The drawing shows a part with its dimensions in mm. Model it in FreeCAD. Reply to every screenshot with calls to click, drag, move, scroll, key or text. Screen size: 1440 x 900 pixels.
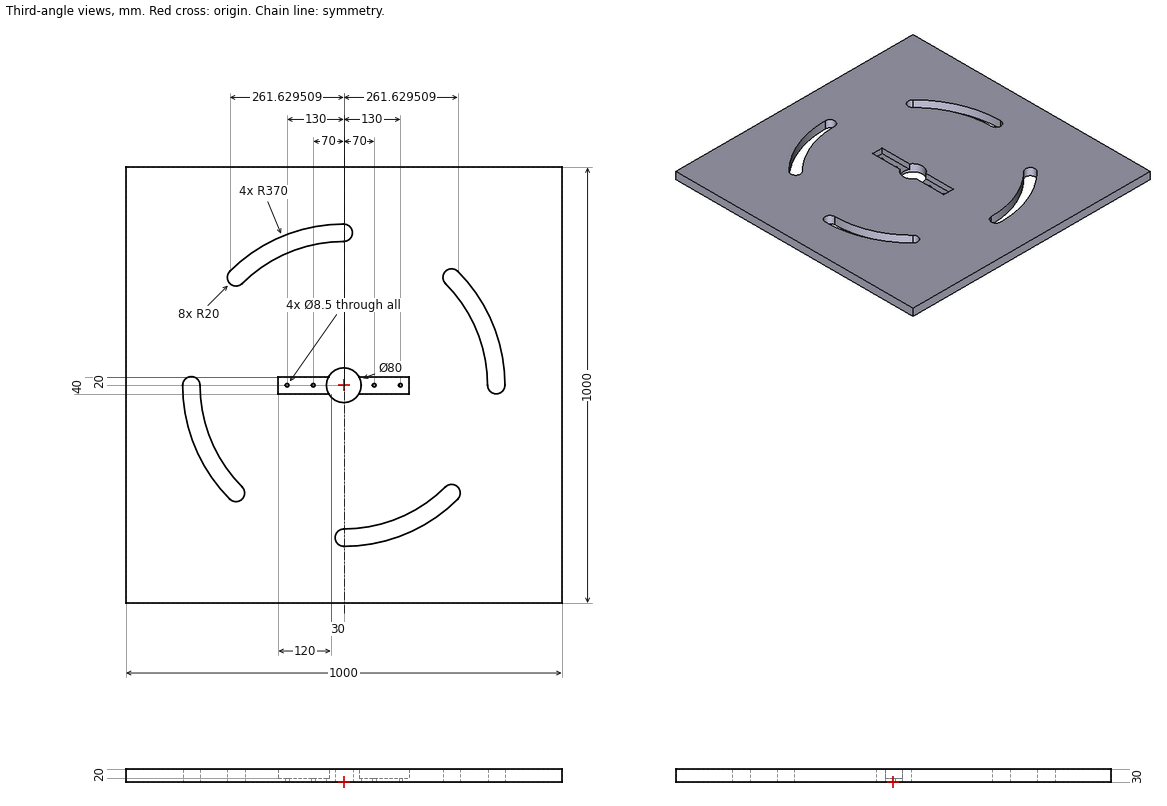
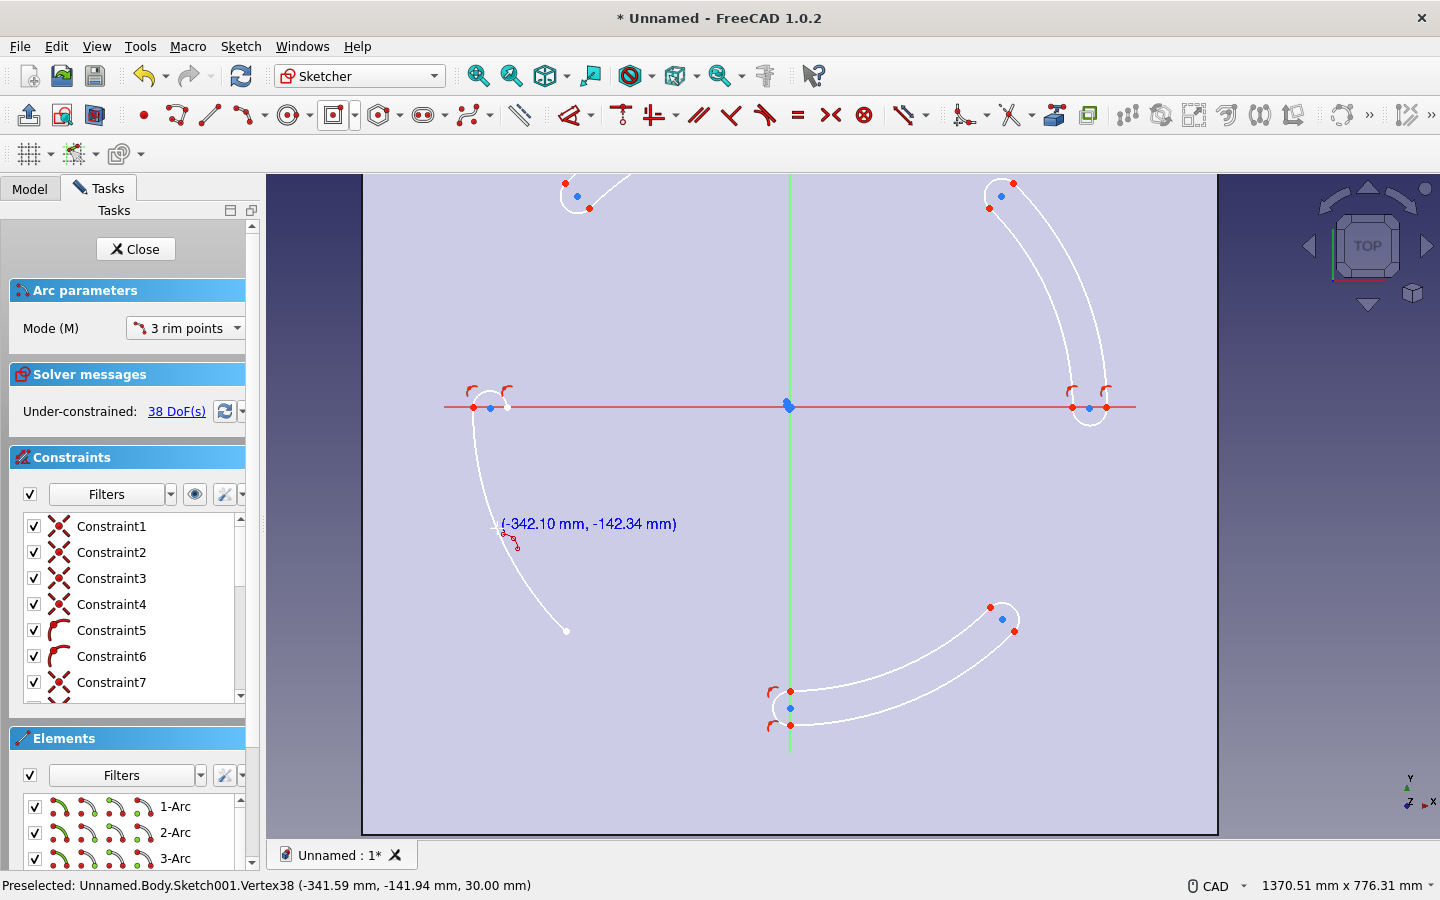
click(566, 632)
click(590, 607)
click(590, 631)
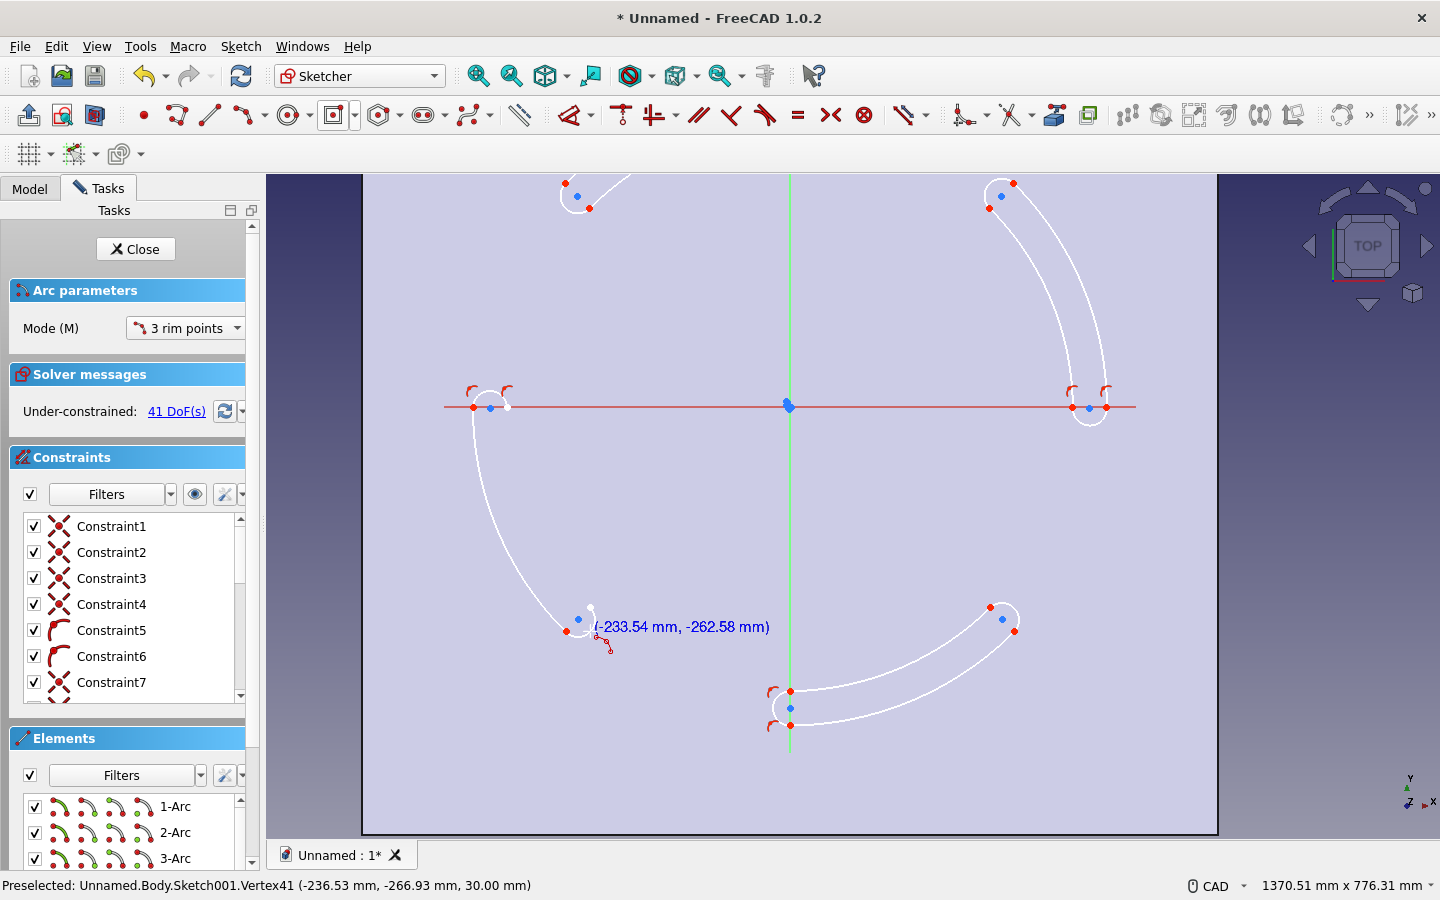
click(590, 608)
click(507, 407)
click(529, 515)
key(Escape)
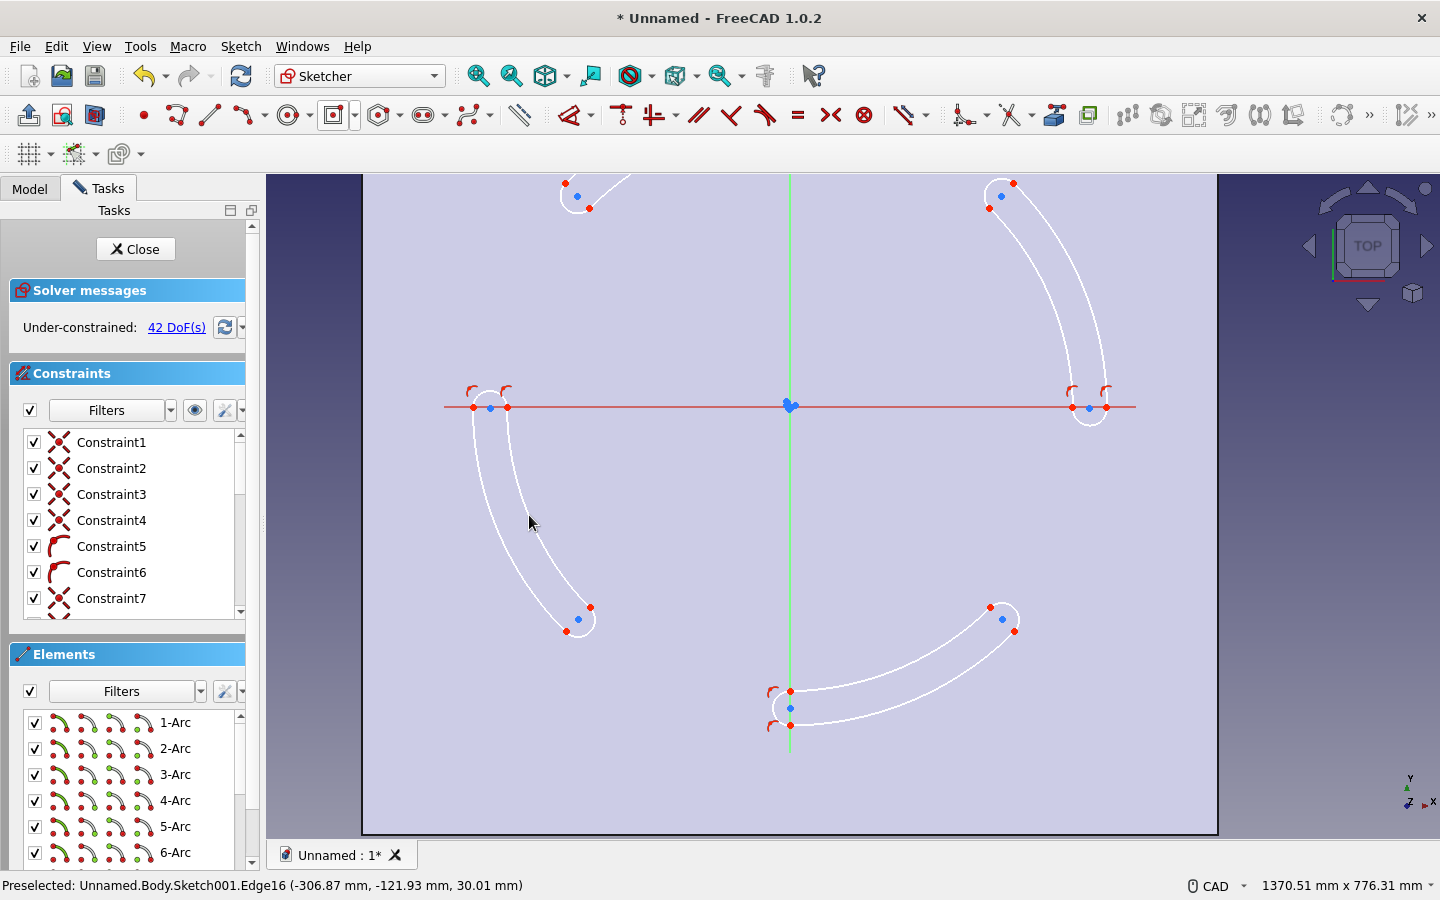
scroll(773, 709, down, 2)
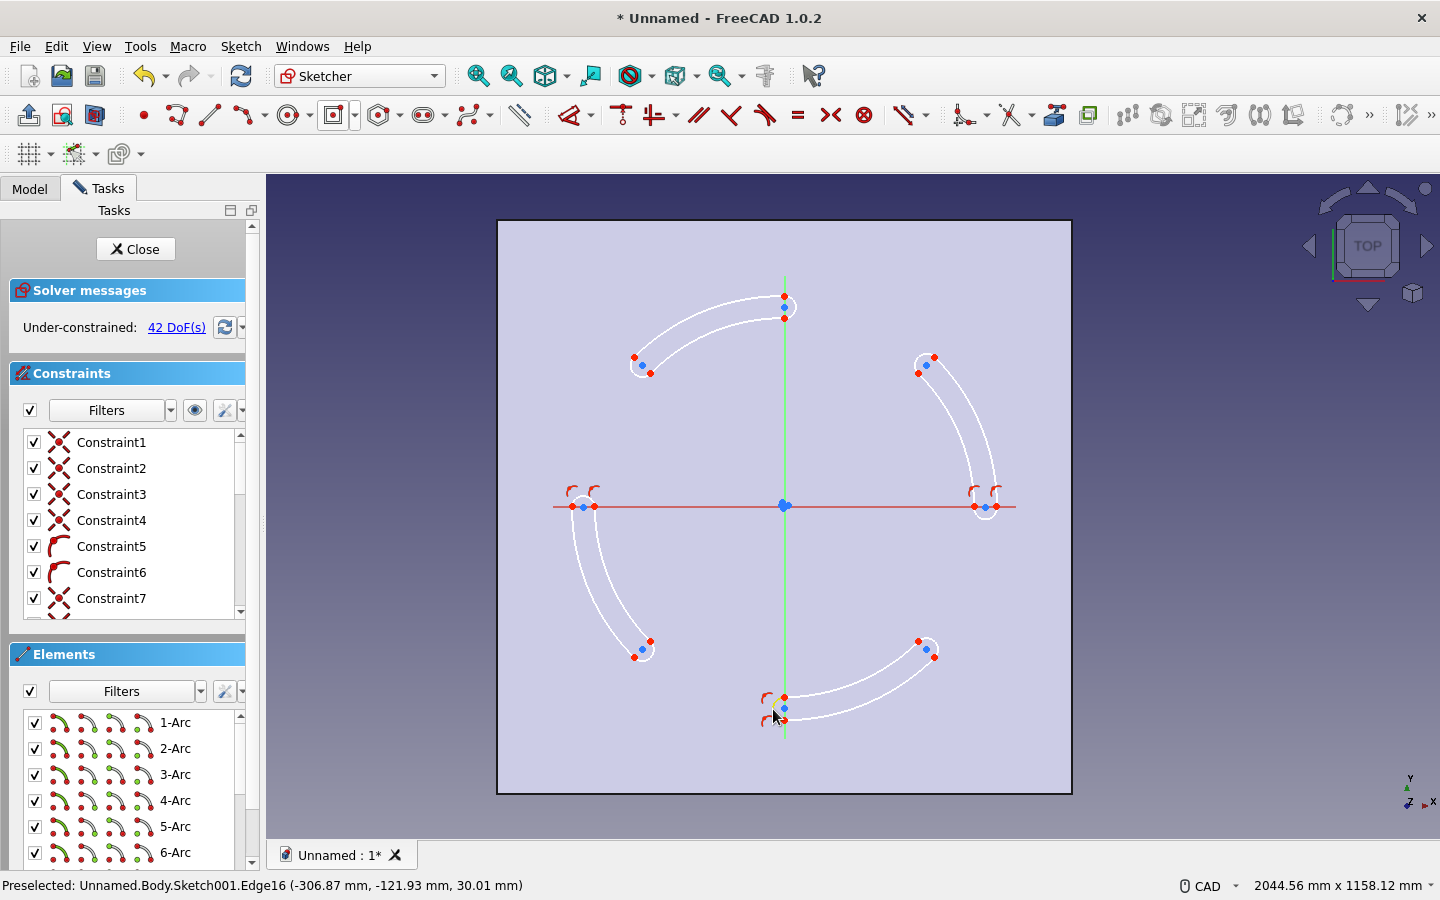
scroll(794, 314, up, 3)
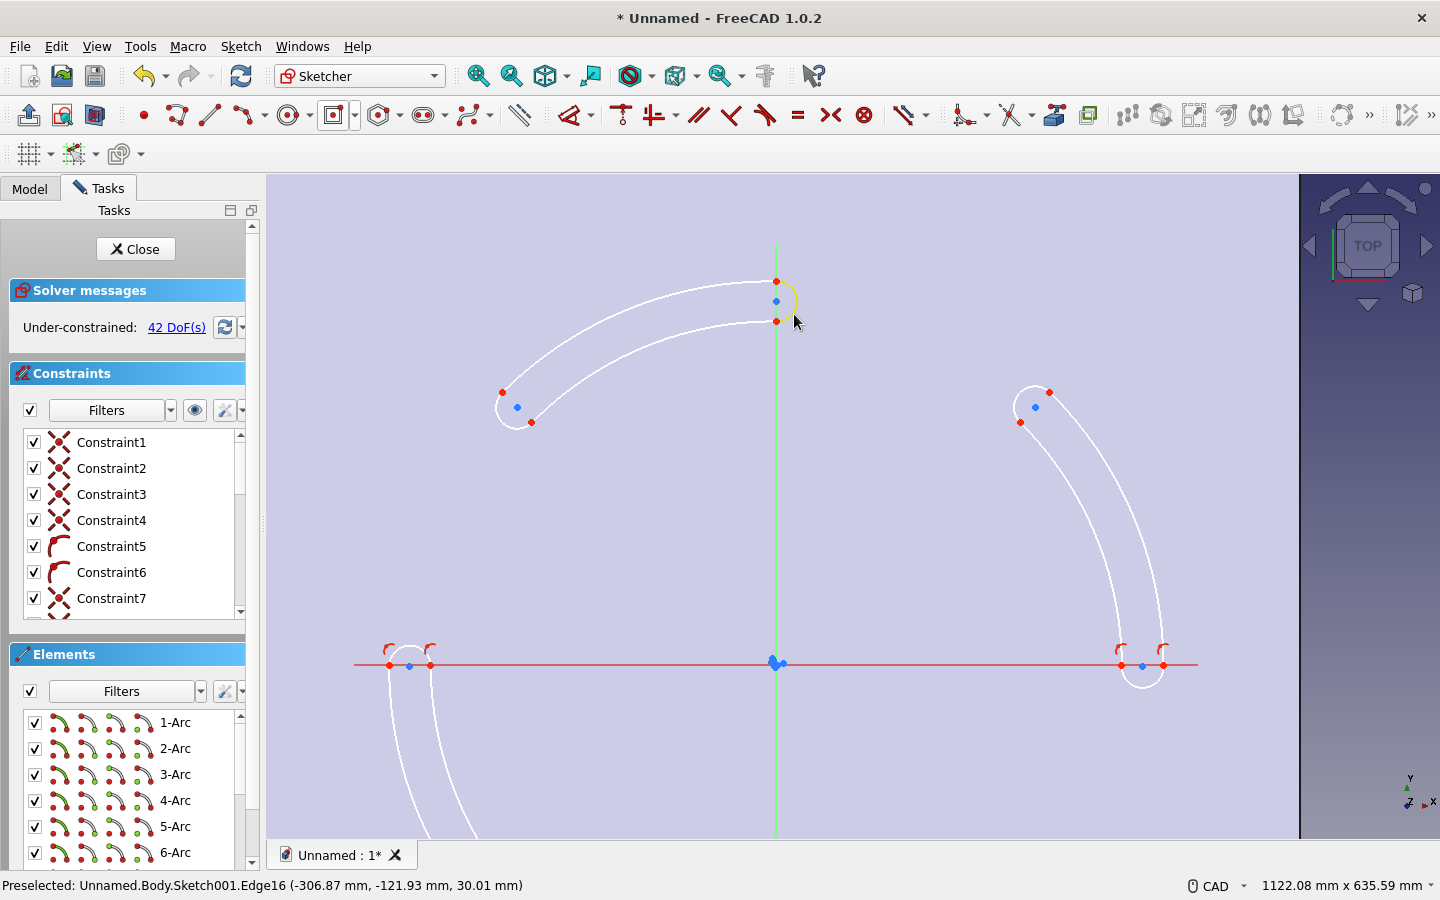
click(793, 313)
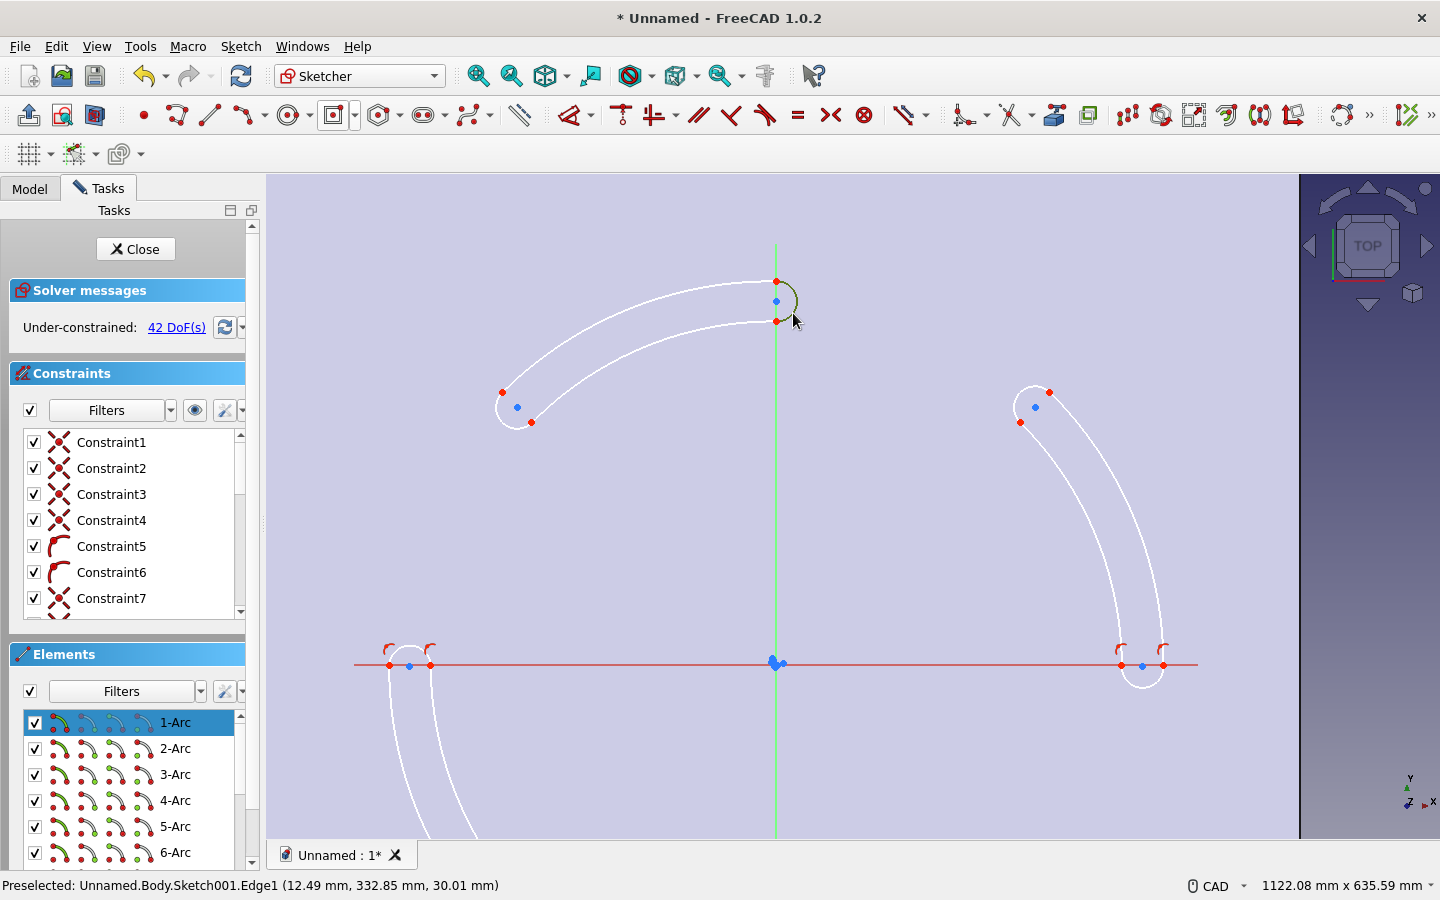
click(686, 291)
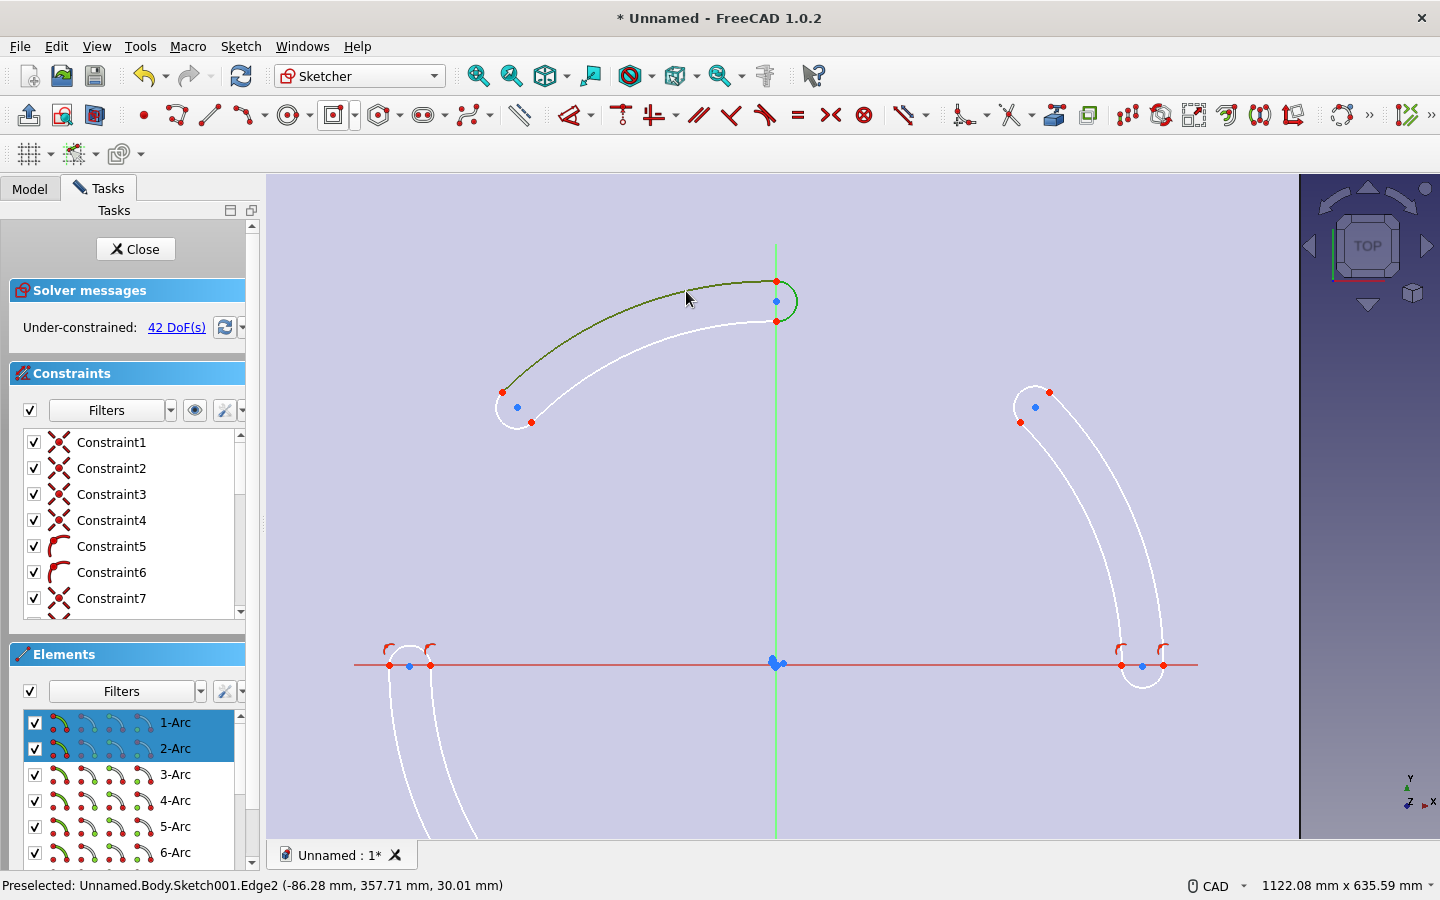
key(t)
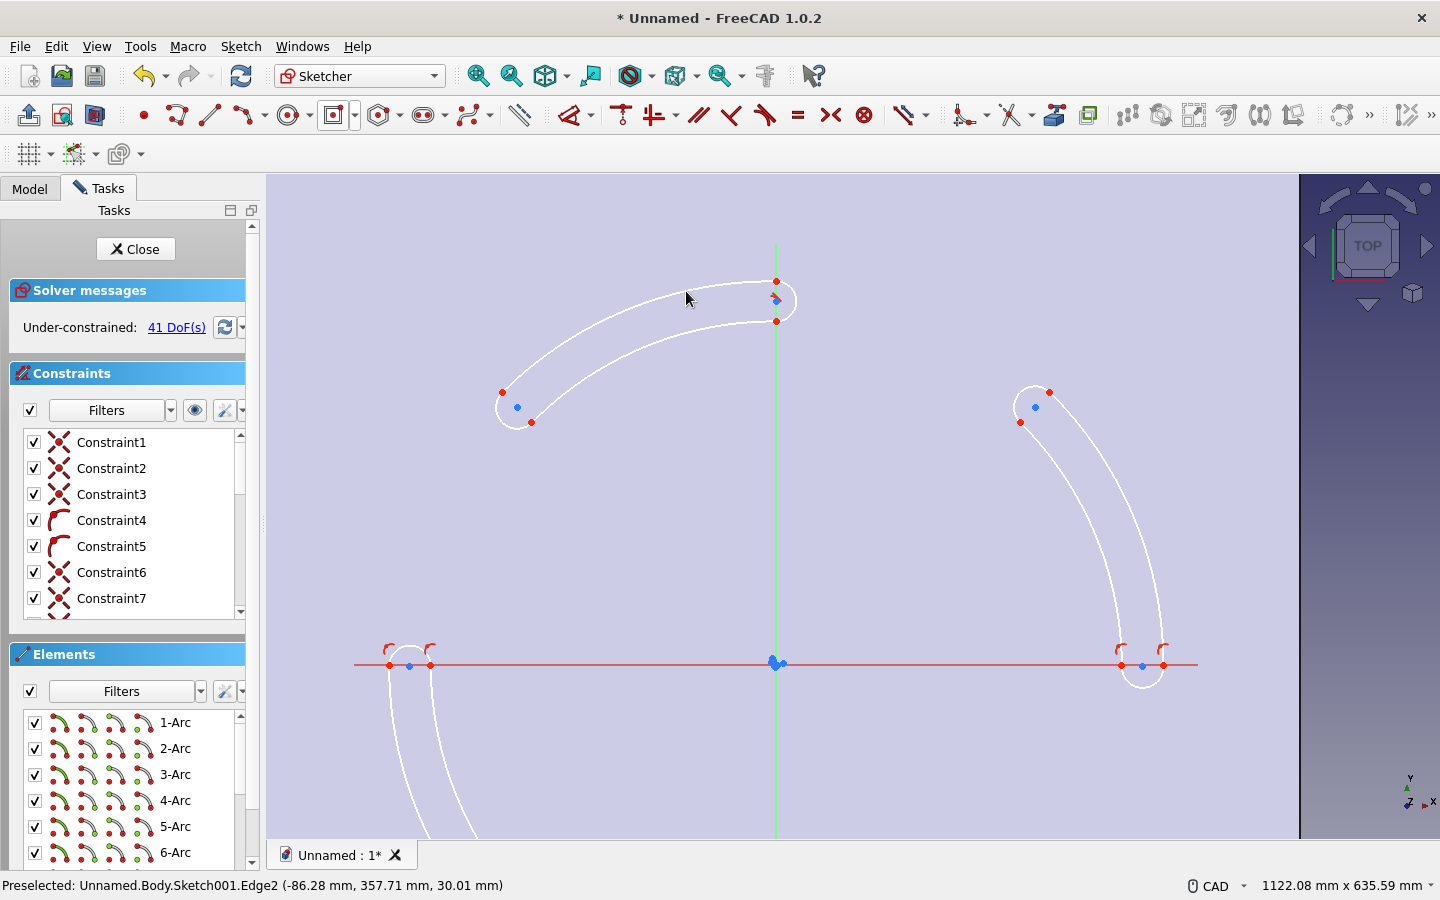
click(792, 313)